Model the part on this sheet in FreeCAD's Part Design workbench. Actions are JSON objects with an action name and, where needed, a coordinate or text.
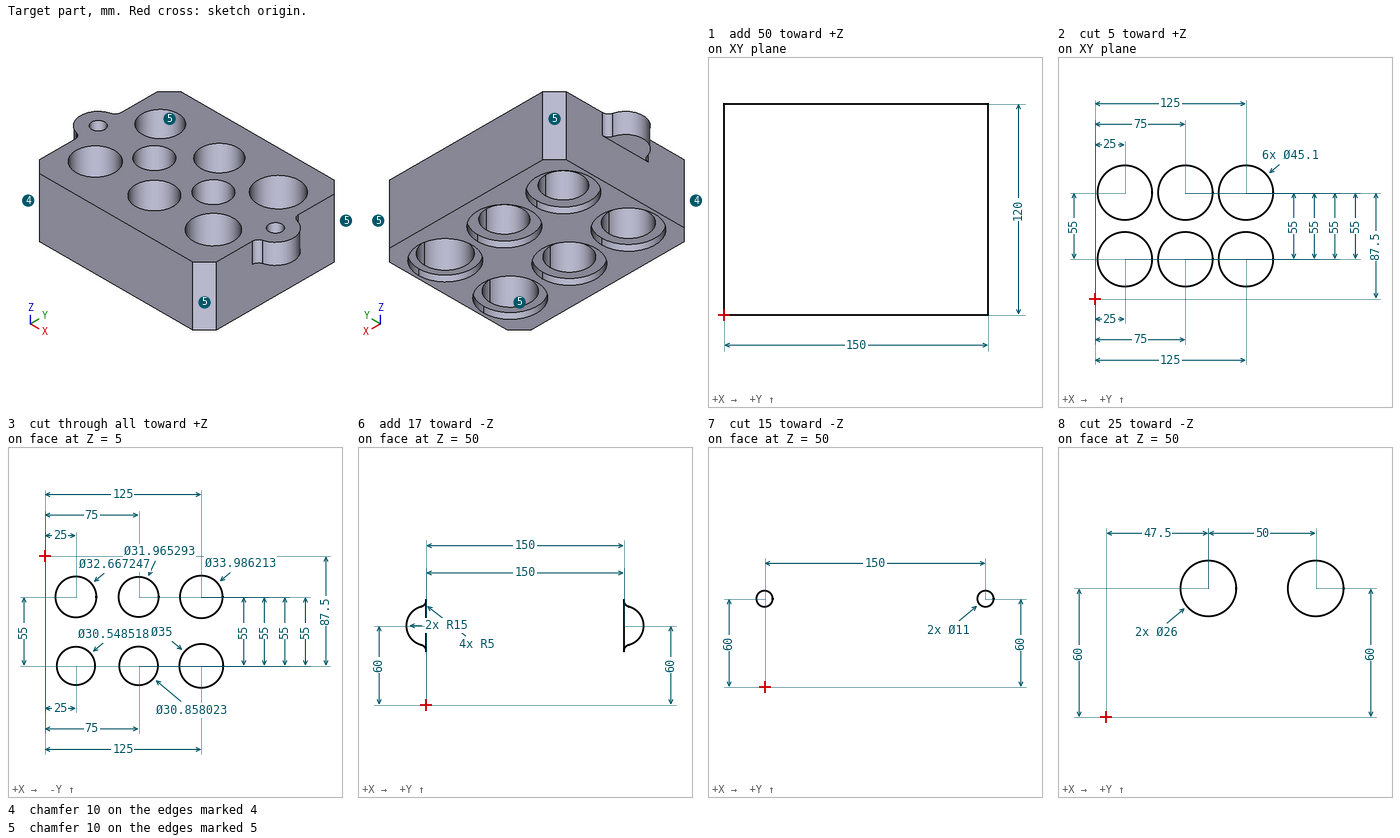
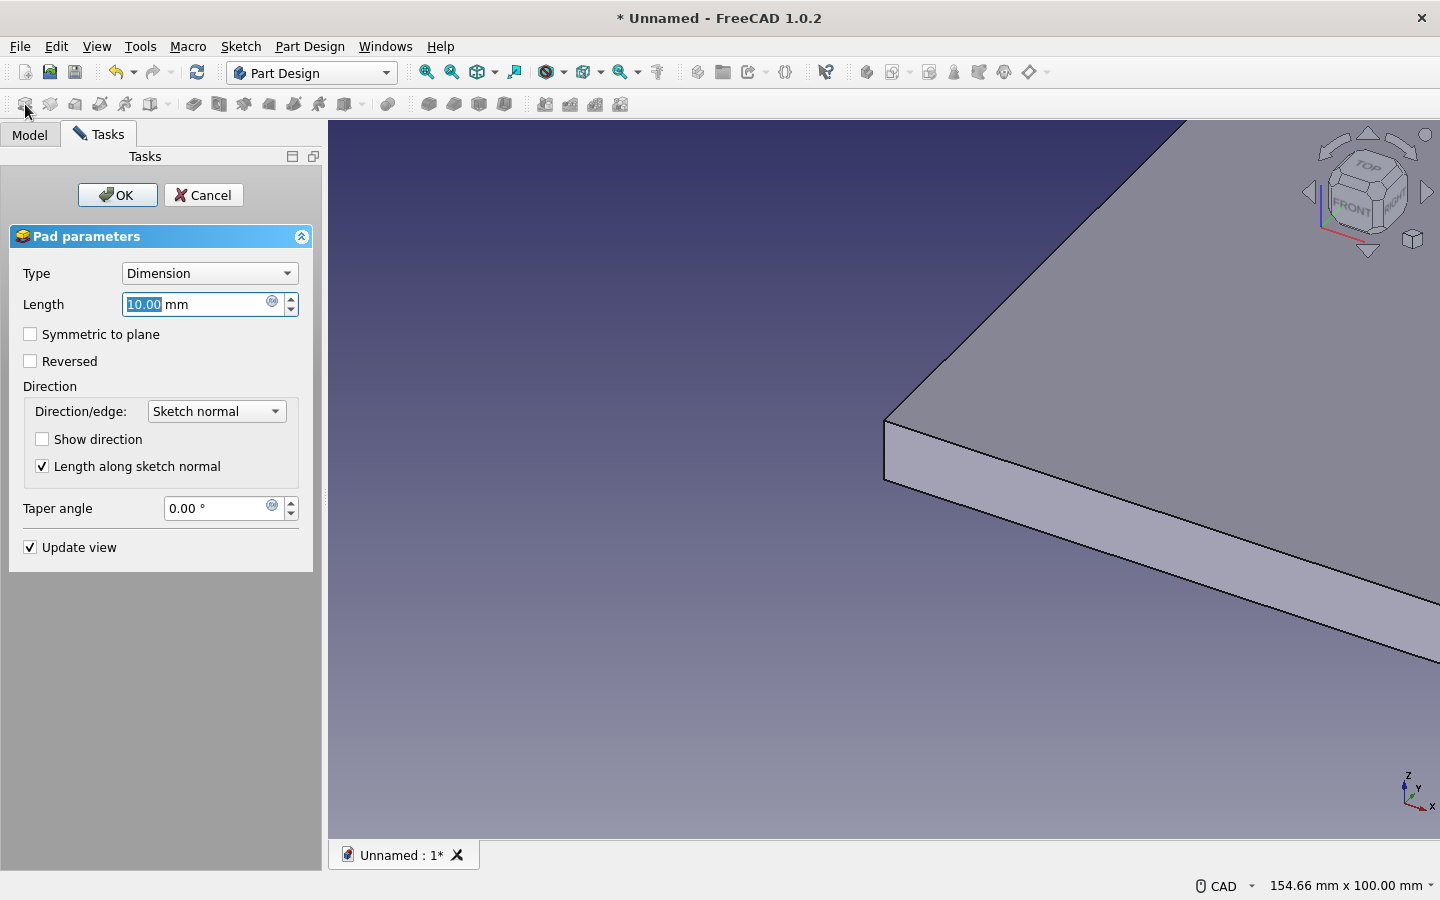
{"action": "type", "text": "50"}
{"action": "key", "text": "Tab"}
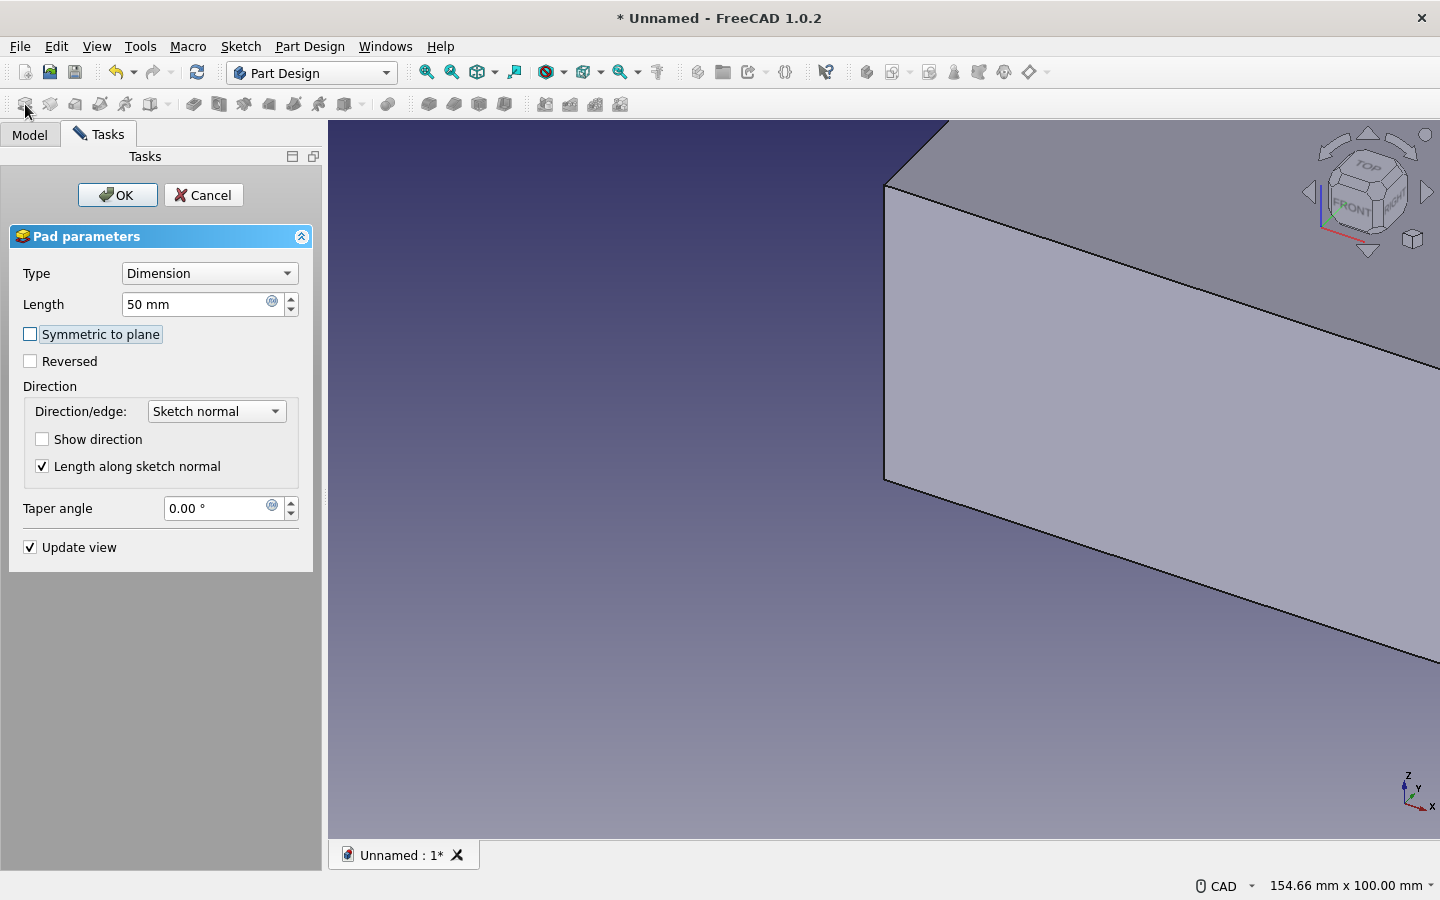
{"action": "left_click", "coordinate": [118, 195]}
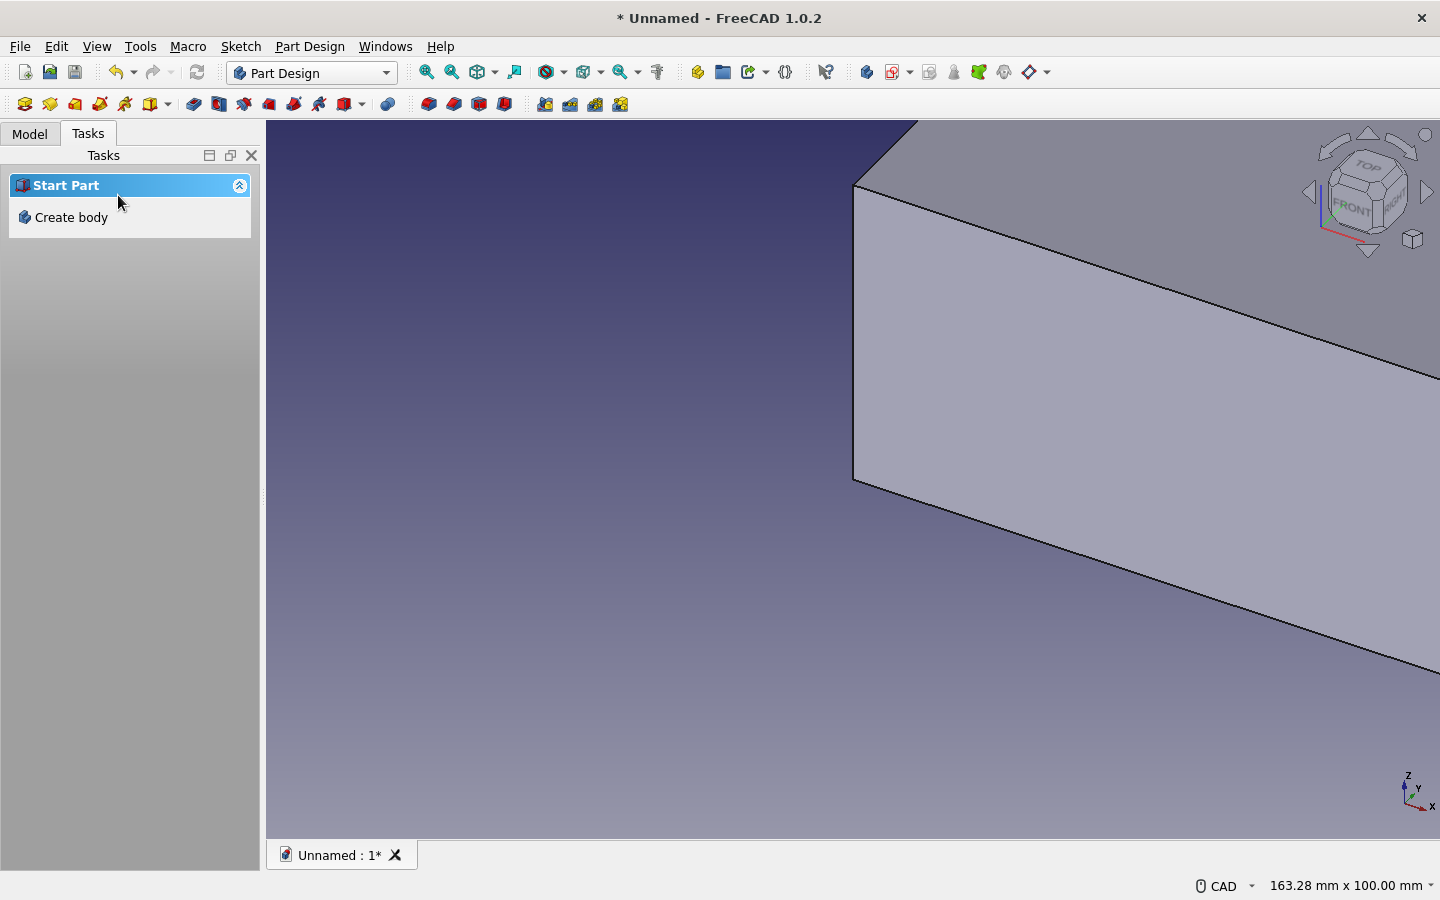
{"action": "left_click", "coordinate": [427, 72]}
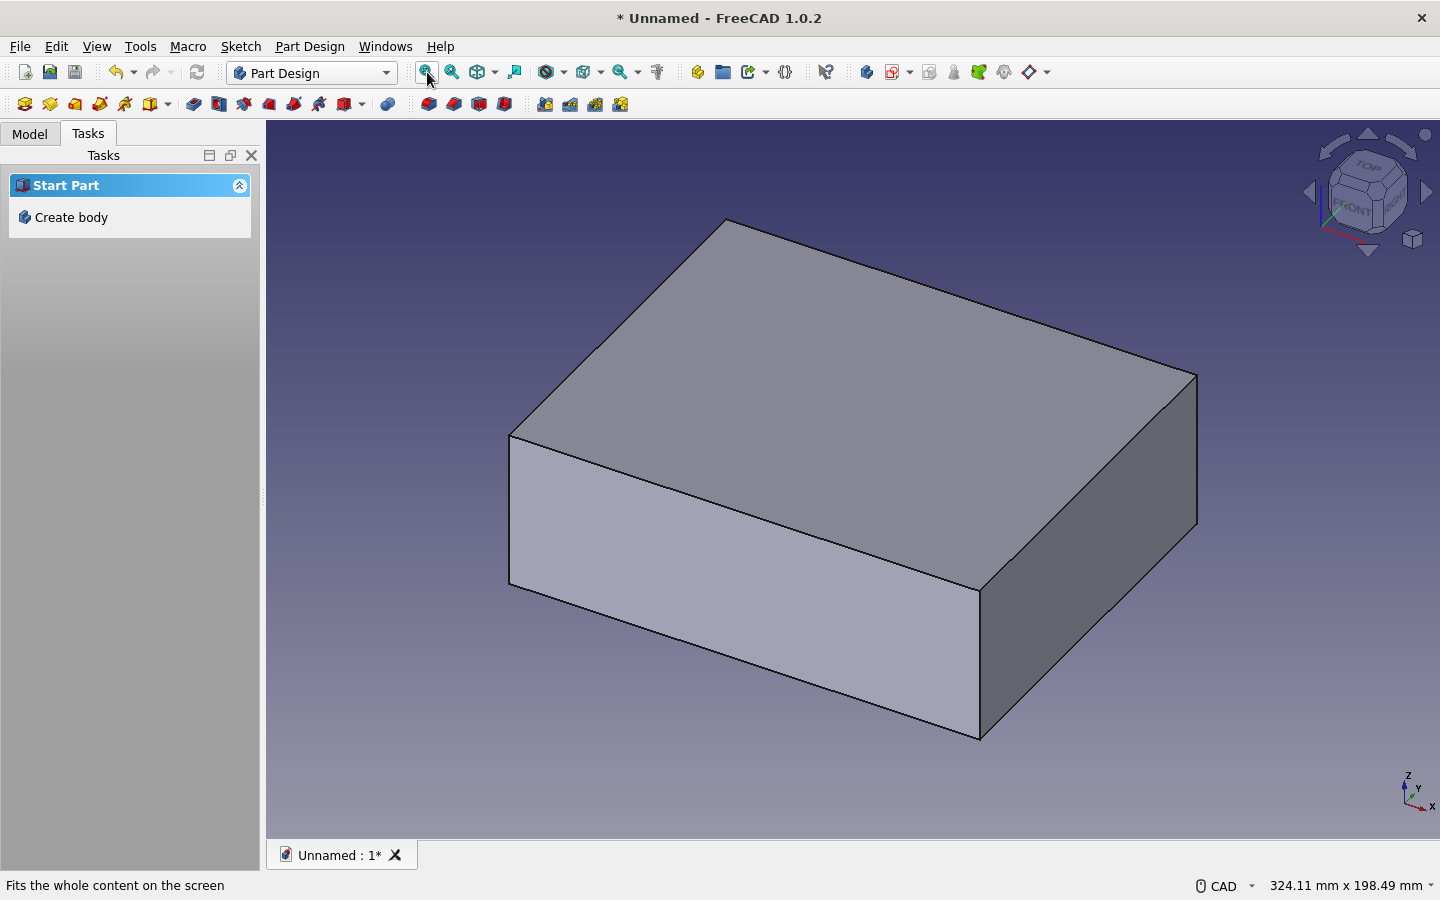
{"action": "left_click", "coordinate": [892, 72]}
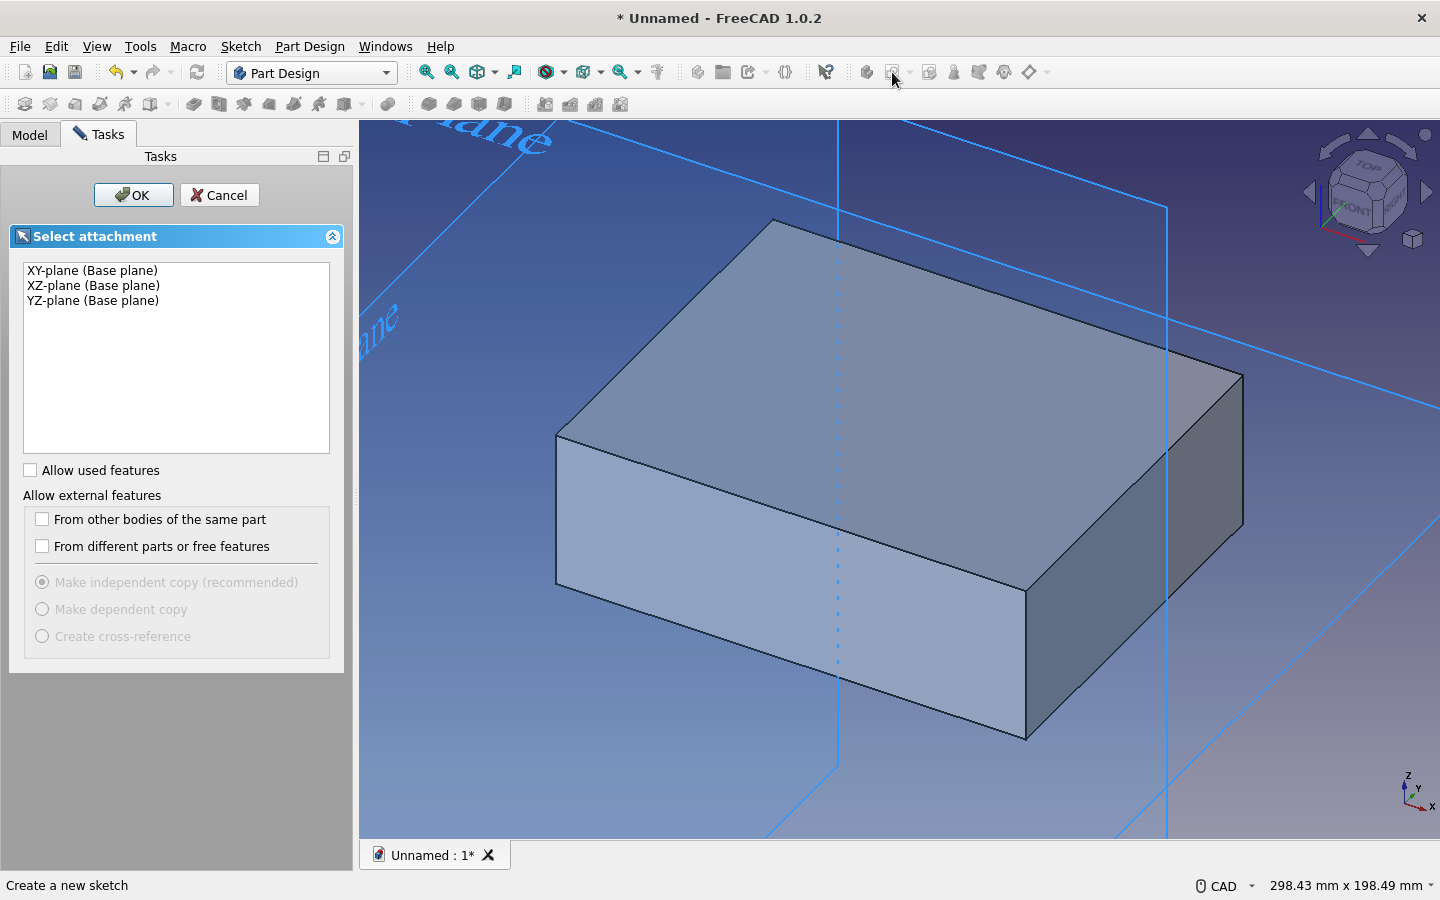
{"action": "left_click", "coordinate": [84, 270]}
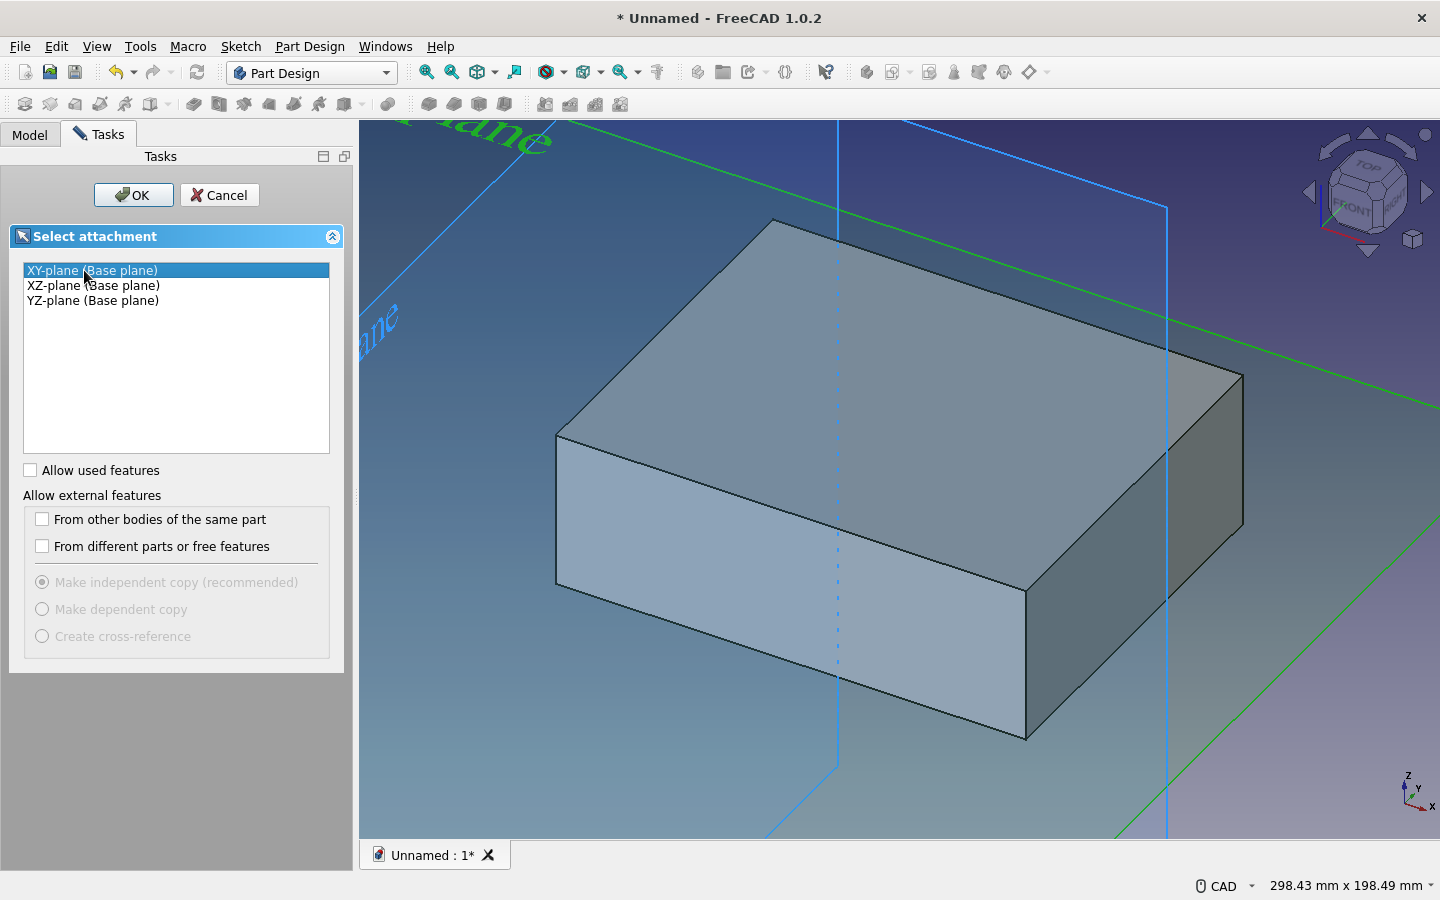
{"action": "left_click", "coordinate": [134, 195]}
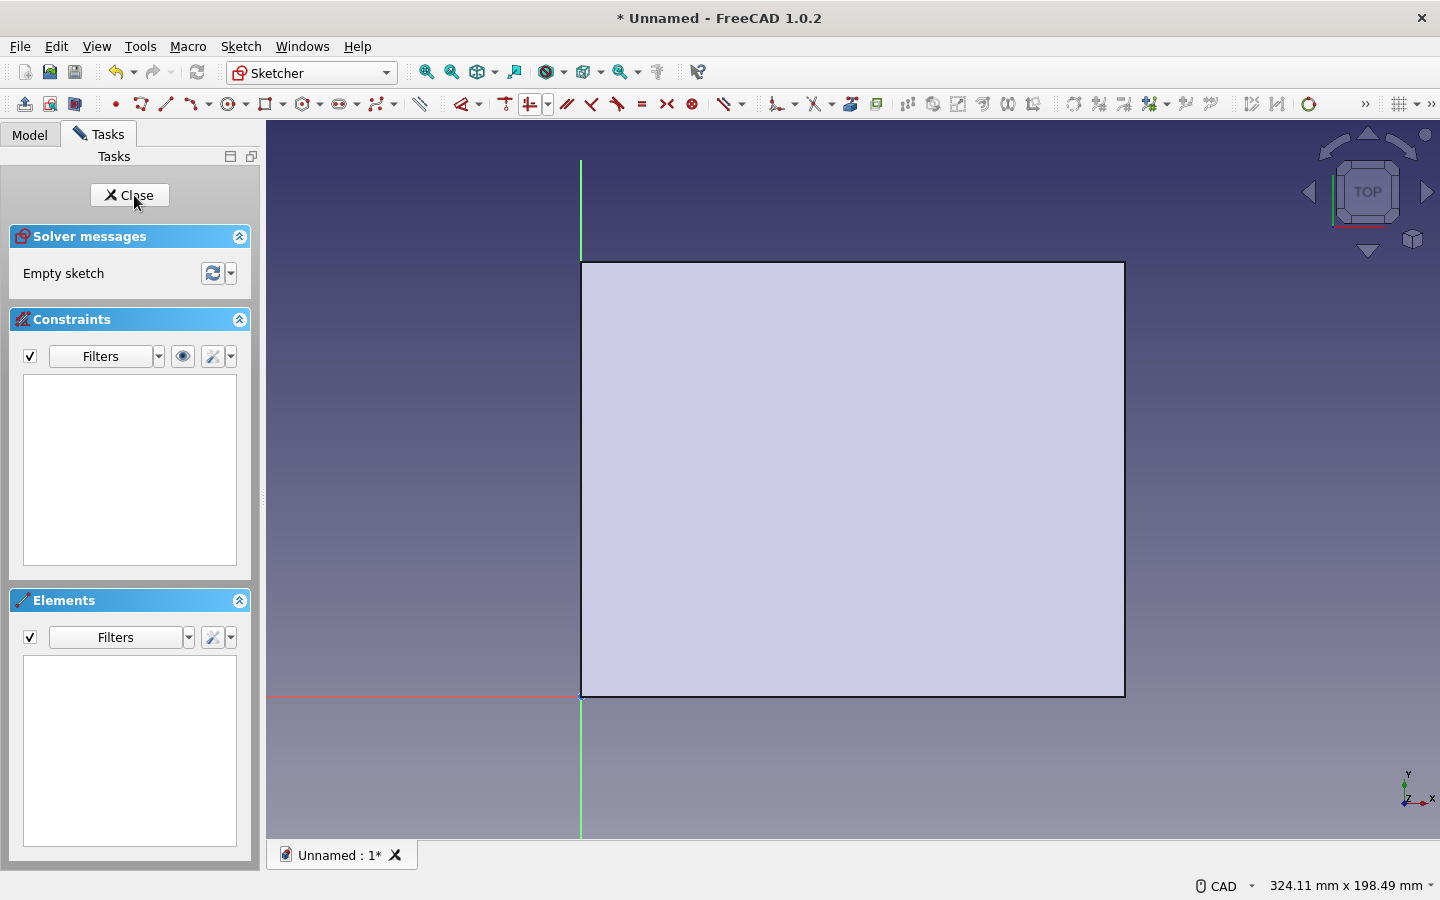
{"action": "left_click", "coordinate": [75, 104]}